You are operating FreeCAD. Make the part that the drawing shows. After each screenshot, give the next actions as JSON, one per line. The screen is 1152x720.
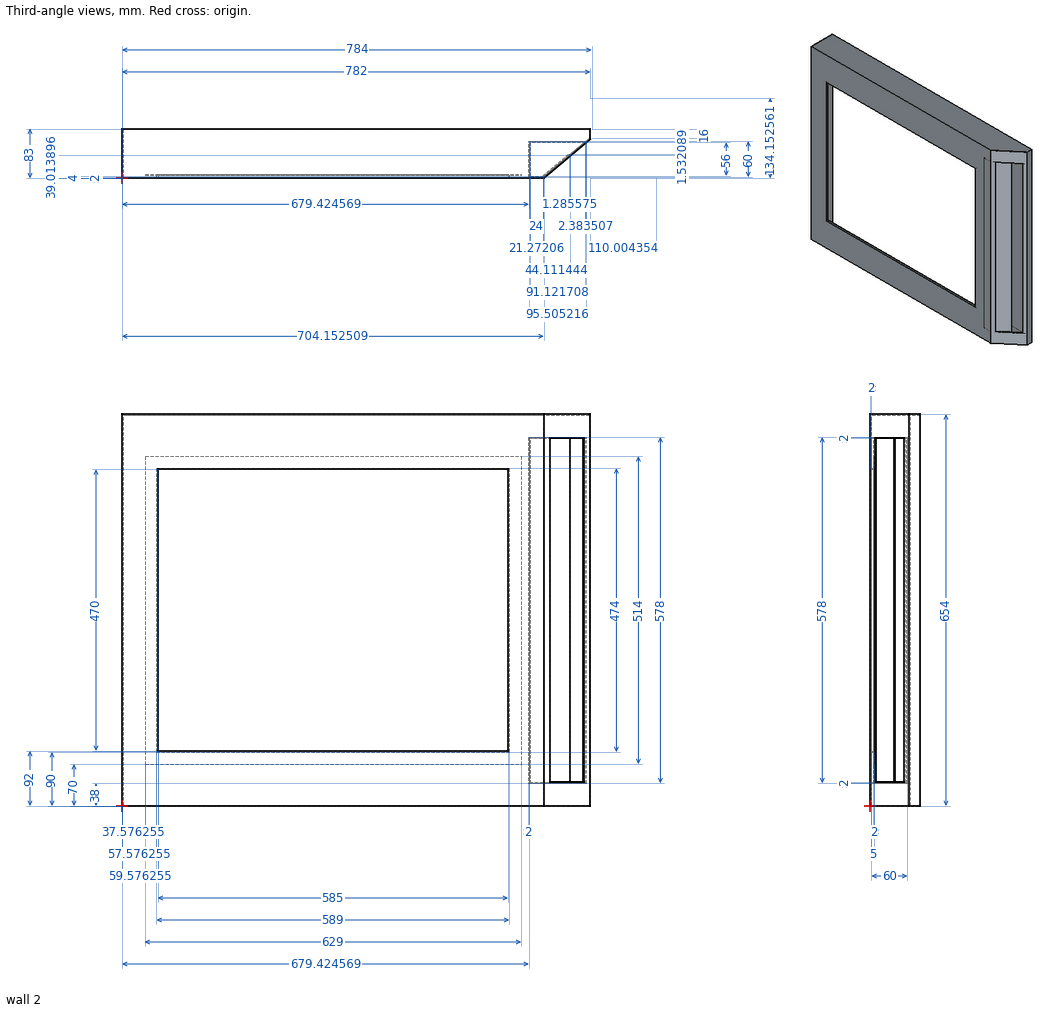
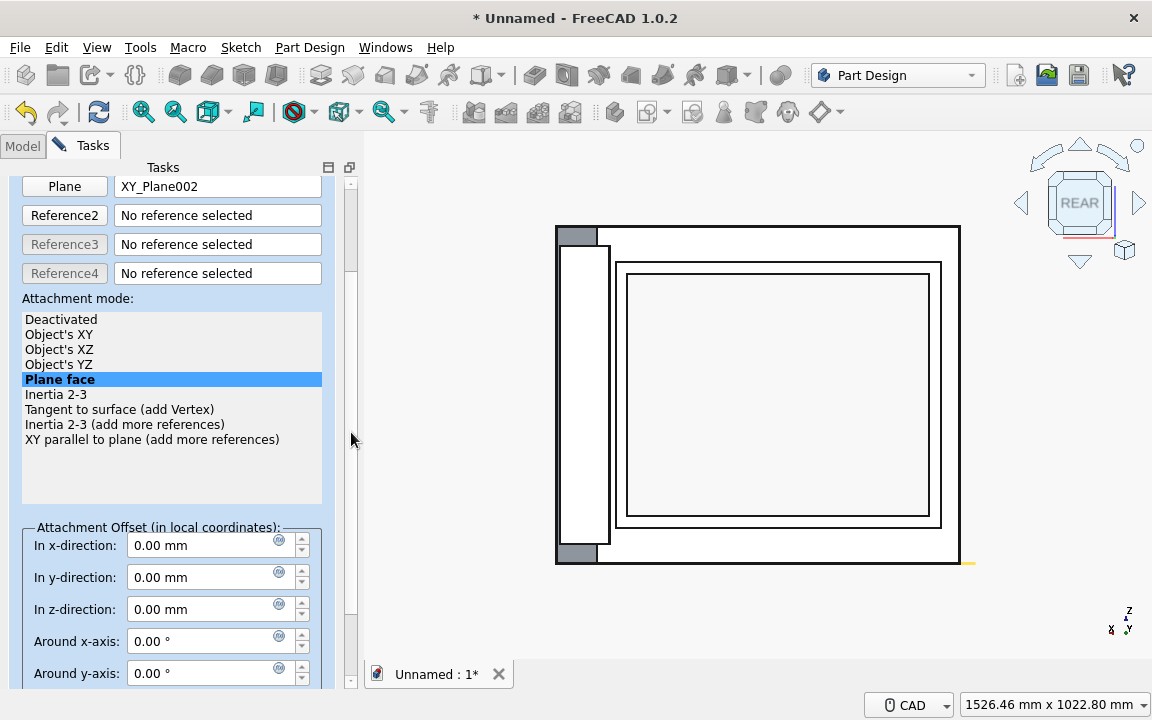
{"action": "triple_click", "coordinate": [210, 609]}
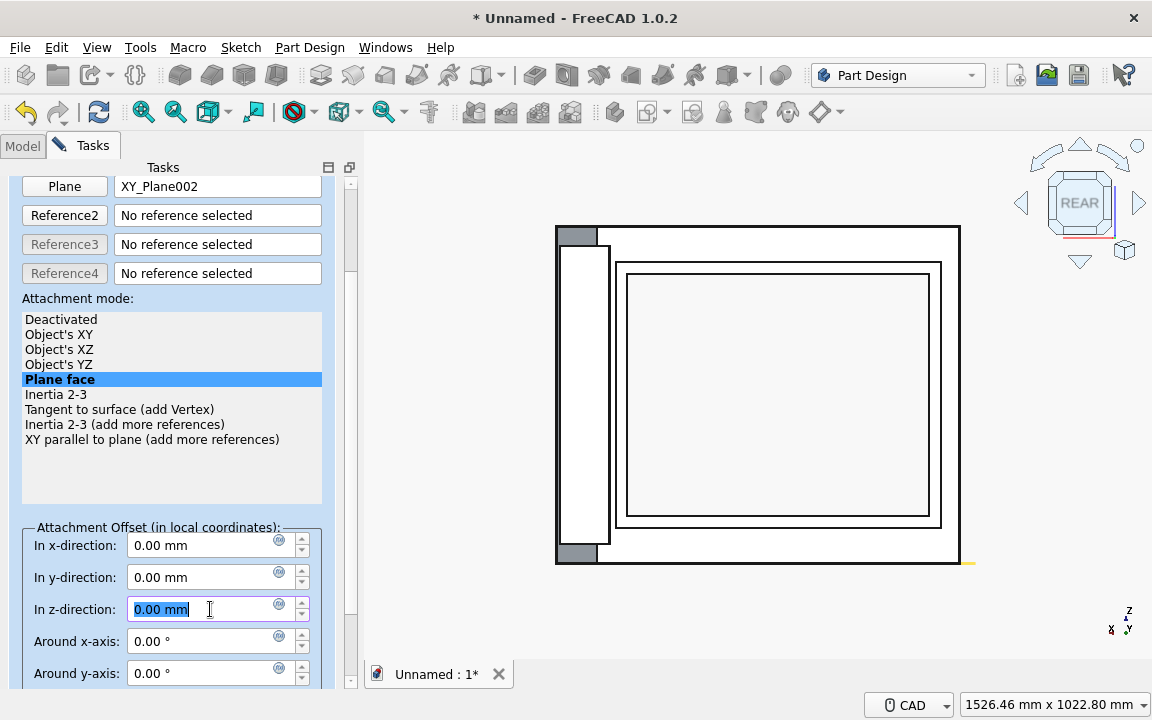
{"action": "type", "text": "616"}
{"action": "key", "text": "Tab"}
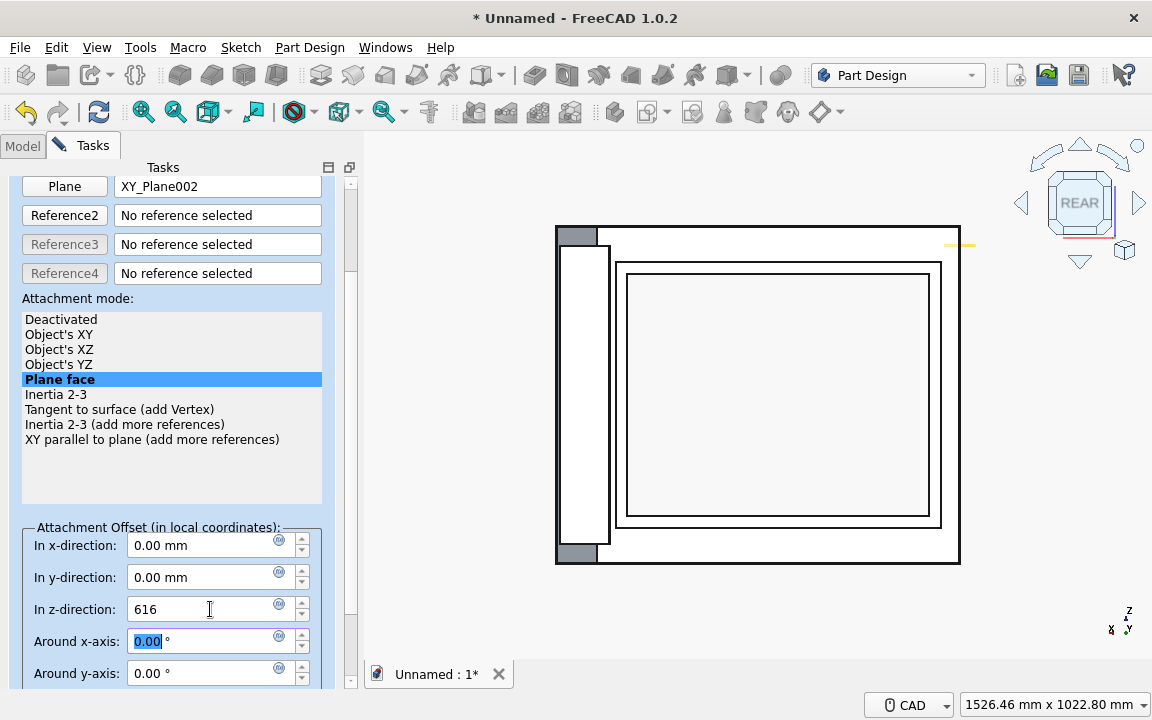
{"action": "scroll", "coordinate": [351, 432], "scroll_direction": "up", "scroll_amount": 3}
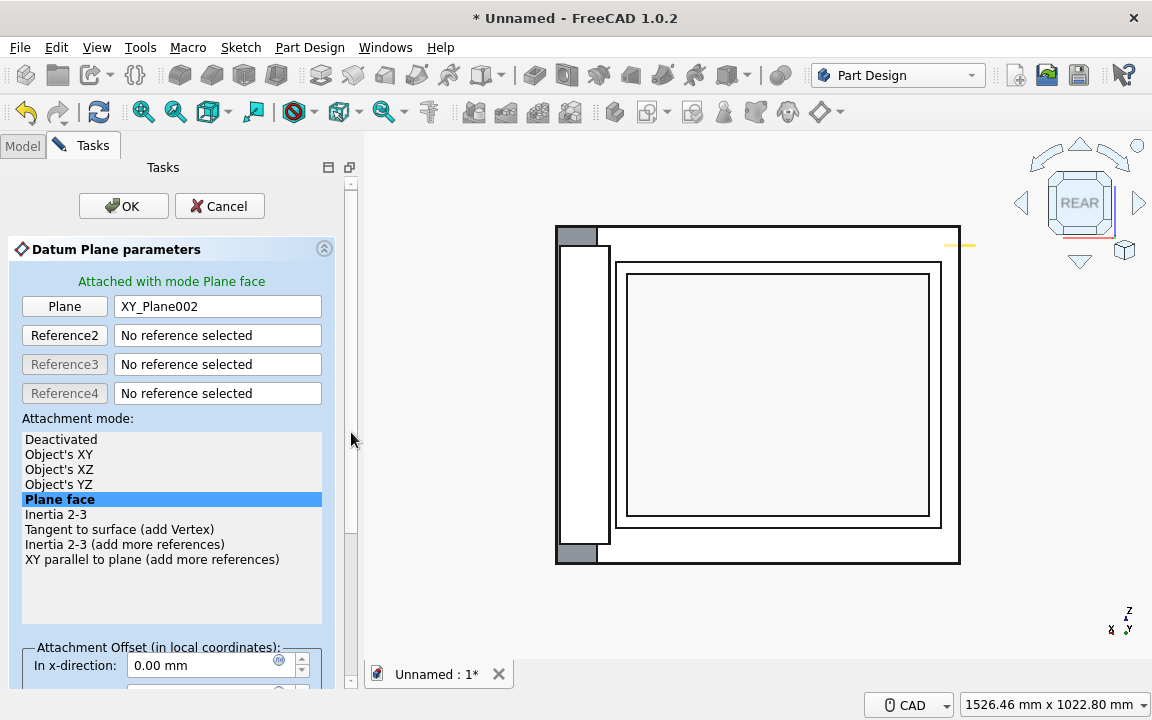
{"action": "left_click", "coordinate": [124, 206]}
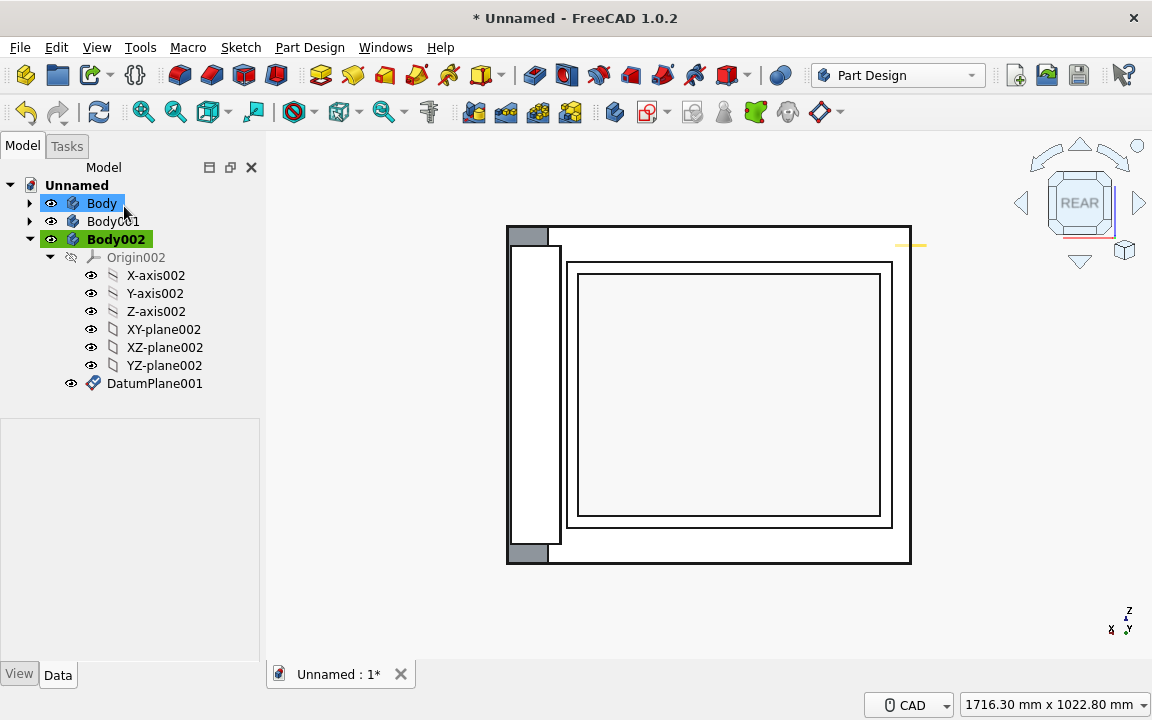
{"action": "left_click", "coordinate": [116, 383]}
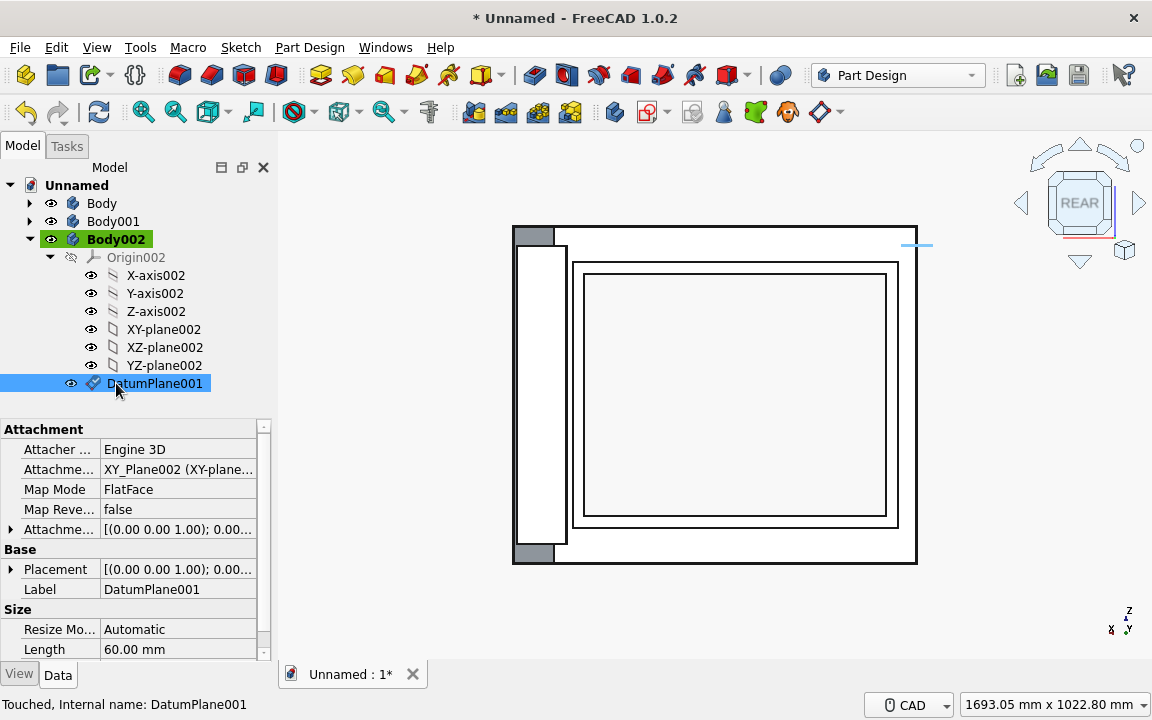
{"action": "left_click", "coordinate": [648, 112]}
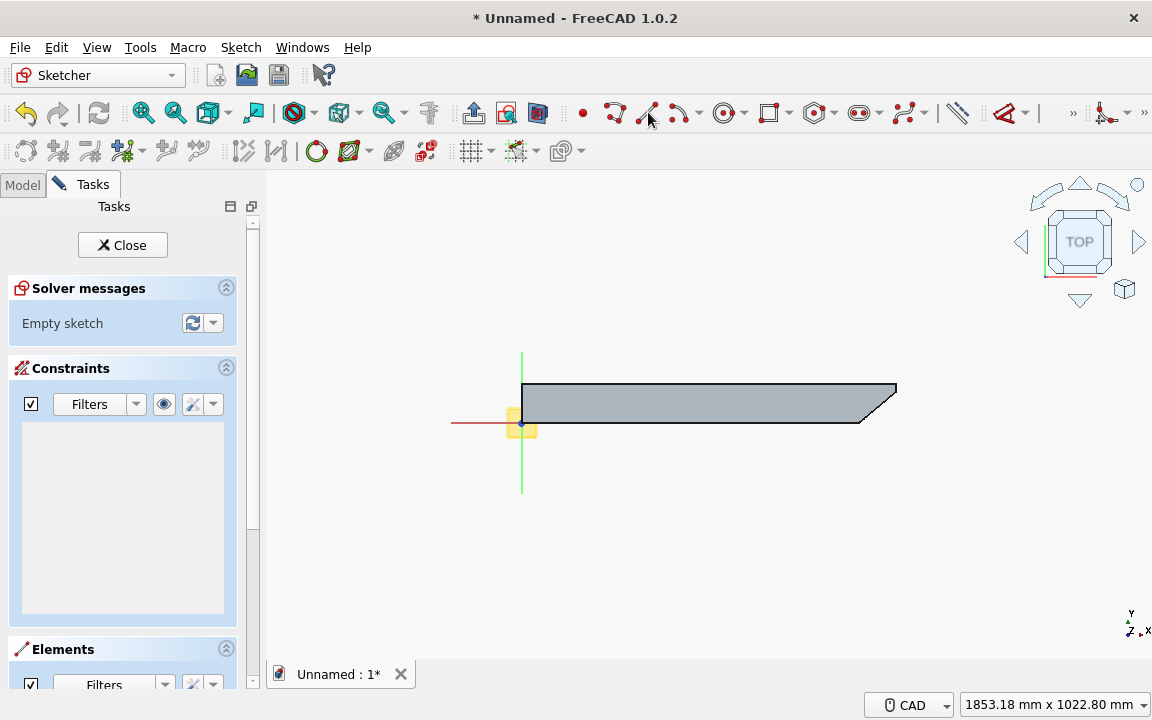
{"action": "scroll", "coordinate": [892, 407], "scroll_direction": "up", "scroll_amount": 12}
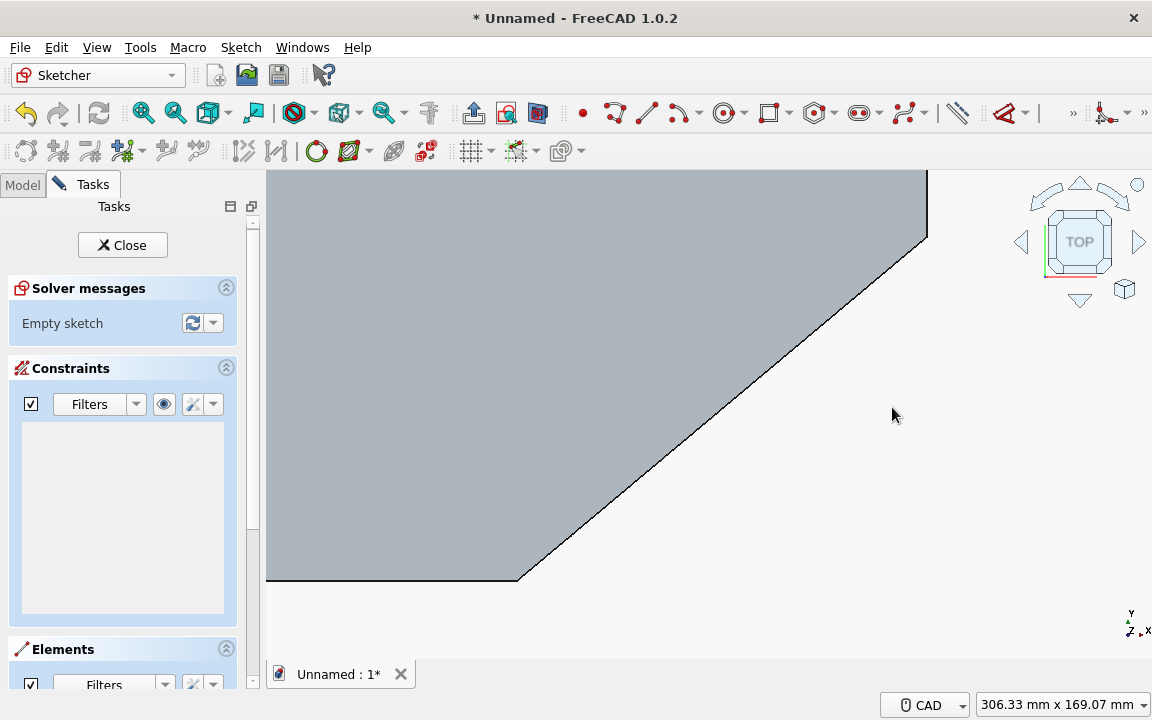
{"action": "left_click", "coordinate": [616, 114]}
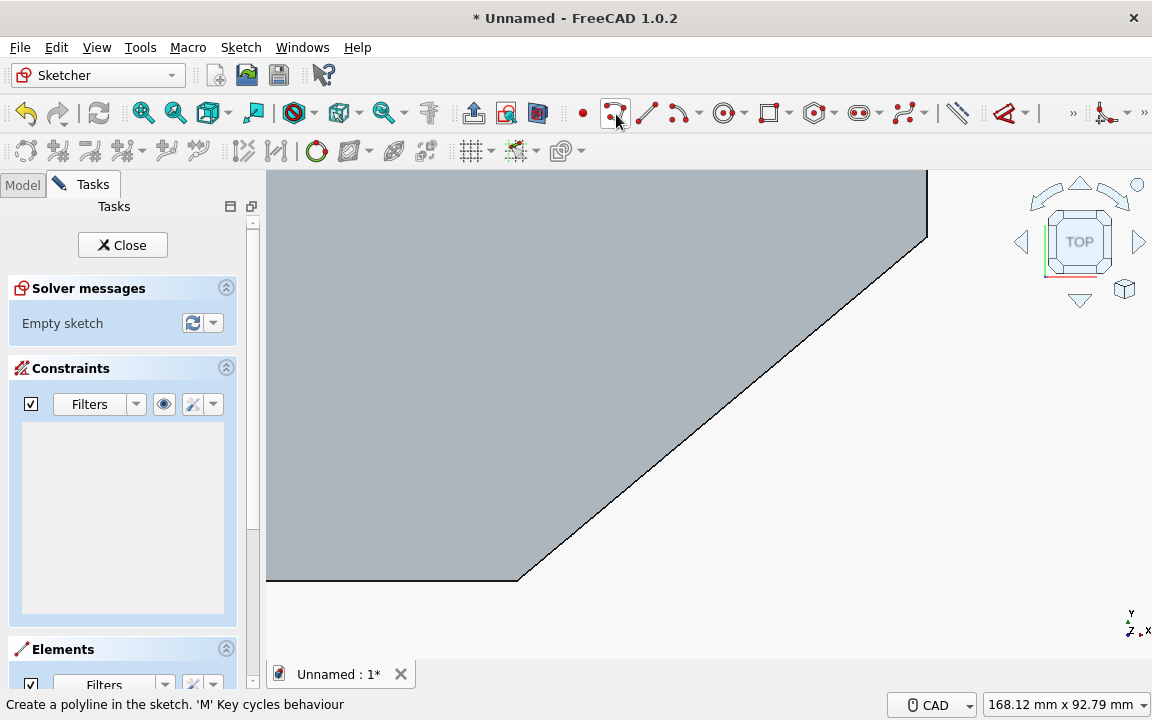
{"action": "scroll", "coordinate": [387, 570], "scroll_direction": "up", "scroll_amount": 3}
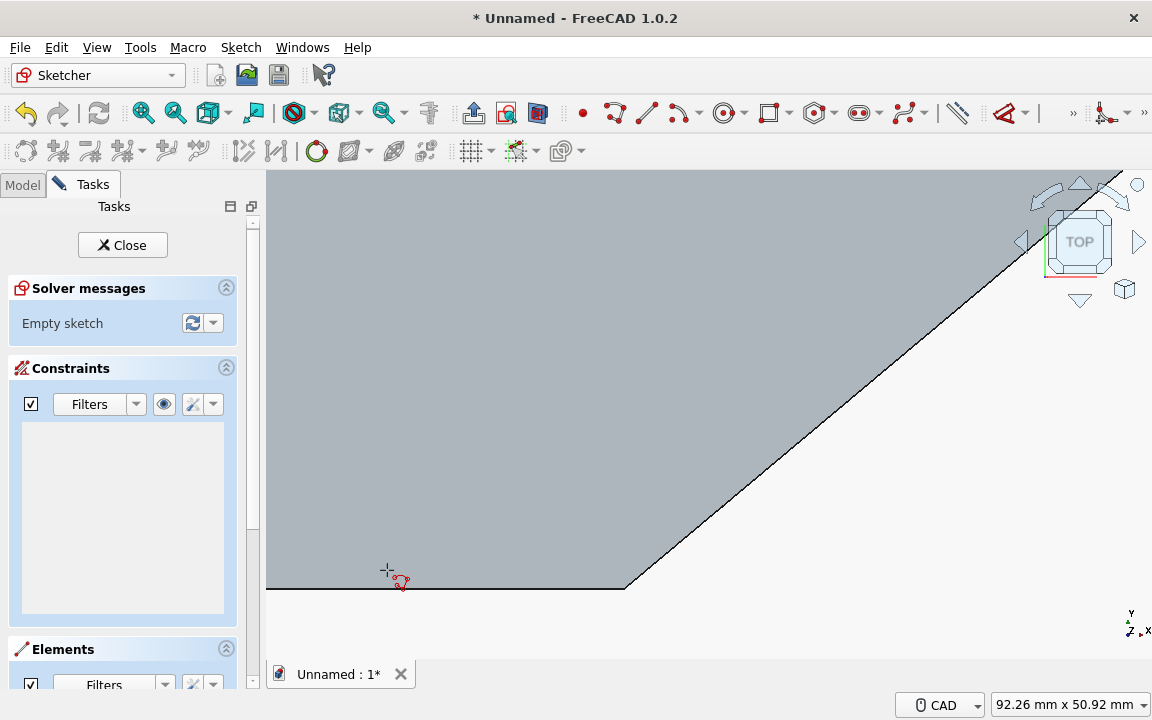
{"action": "left_click", "coordinate": [386, 570]}
{"action": "left_click", "coordinate": [617, 570]}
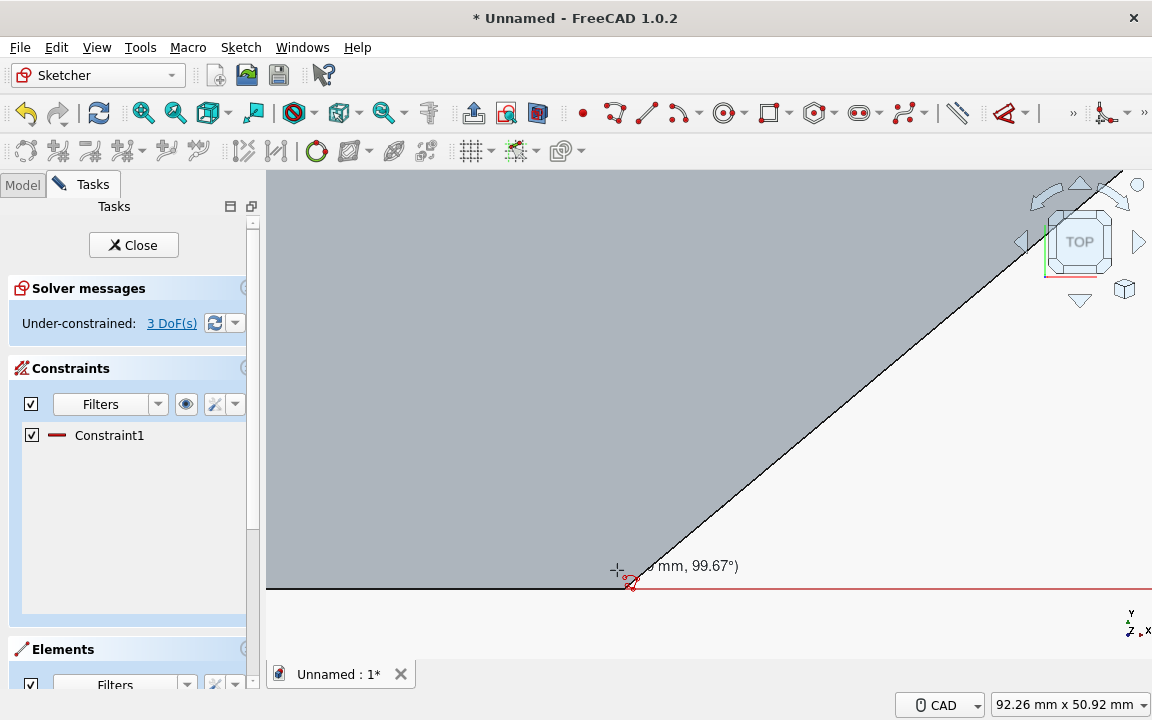
{"action": "scroll", "coordinate": [392, 576], "scroll_direction": "down", "scroll_amount": 3}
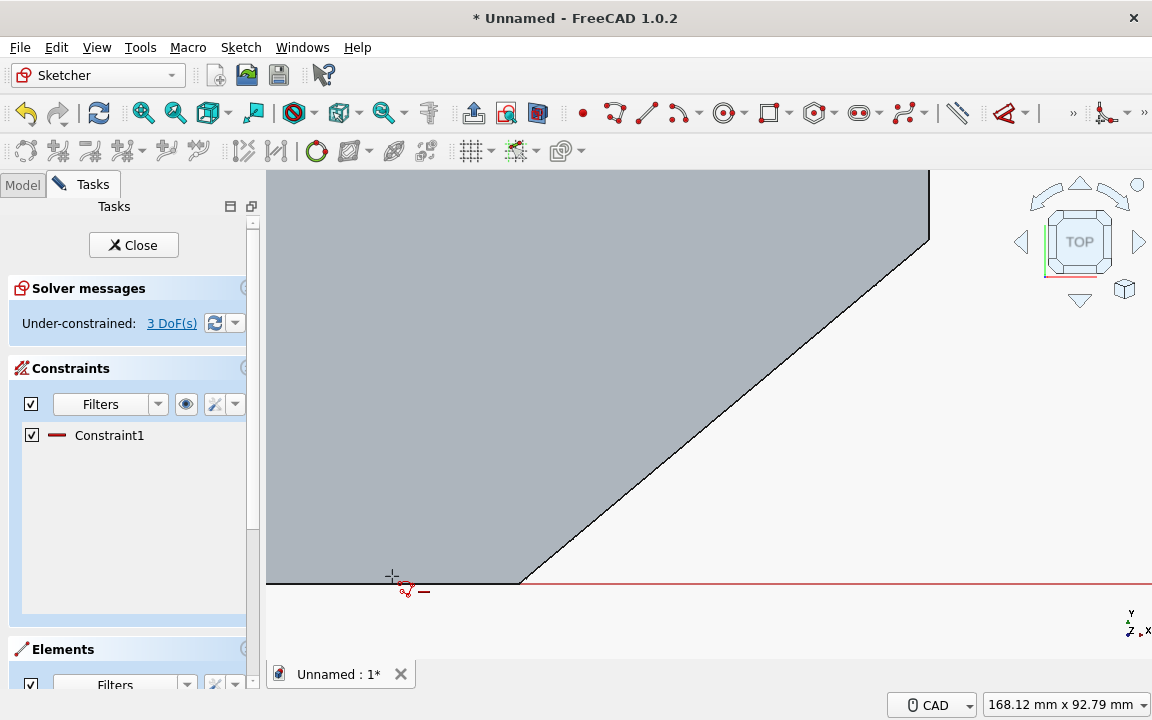
{"action": "left_click", "coordinate": [892, 257]}
{"action": "left_click", "coordinate": [389, 257]}